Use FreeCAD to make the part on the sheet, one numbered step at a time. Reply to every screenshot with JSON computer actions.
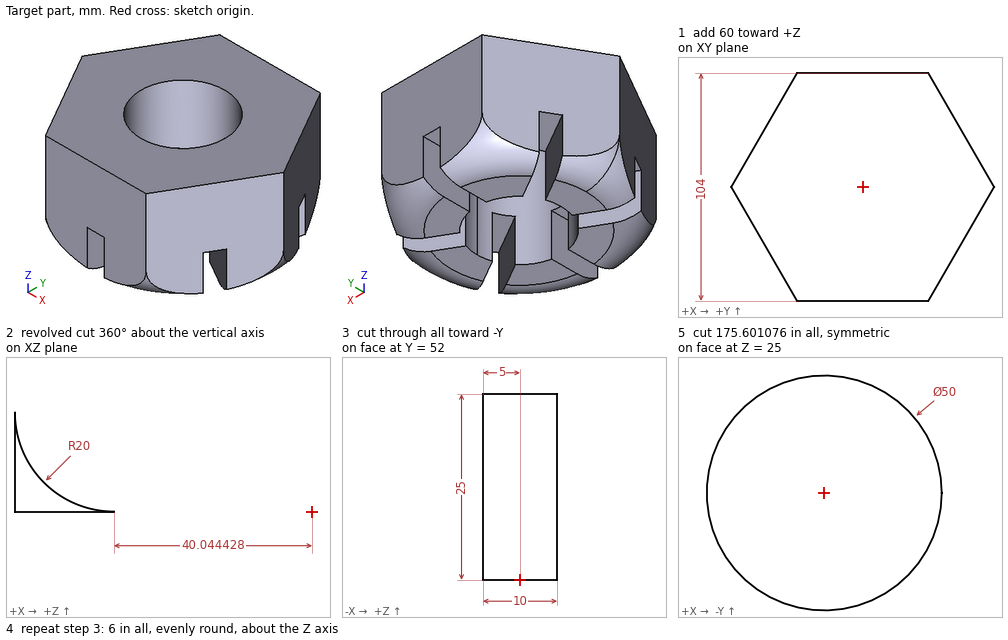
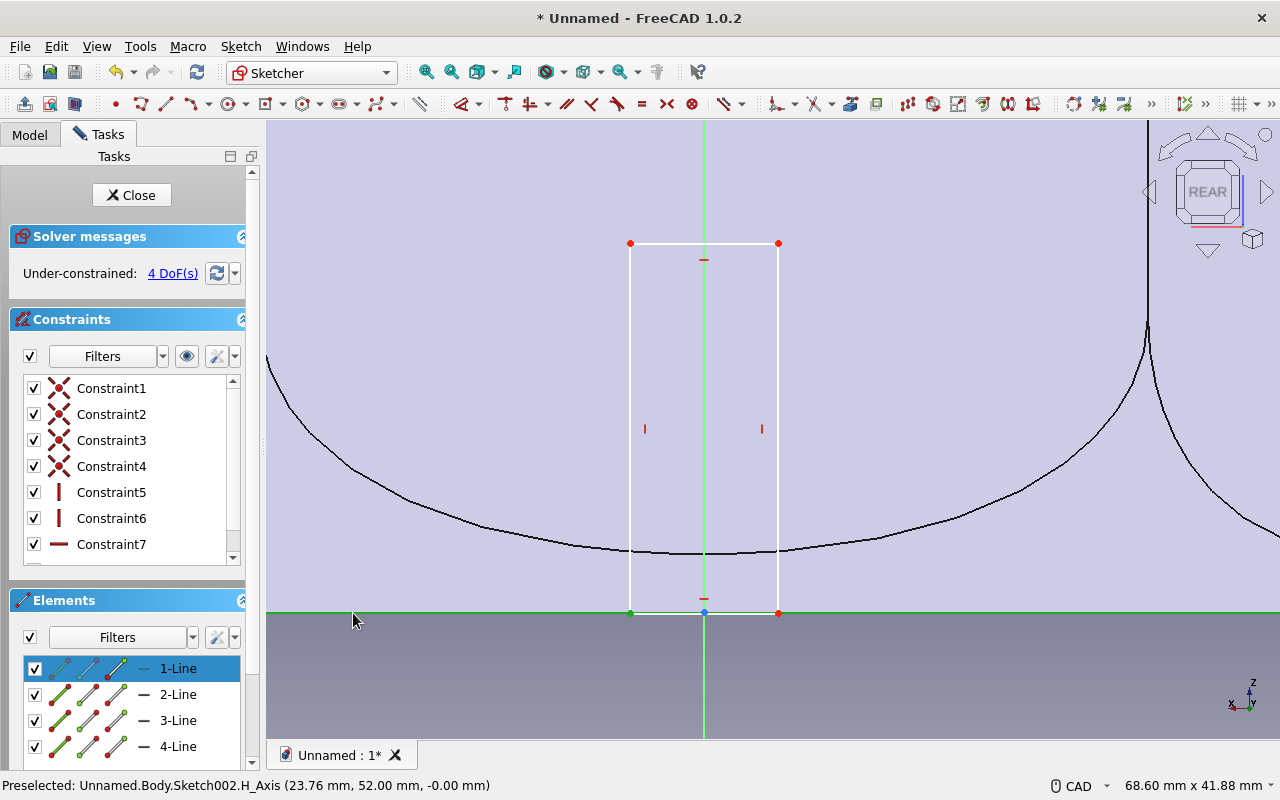
{"action": "left_click", "coordinate": [505, 104]}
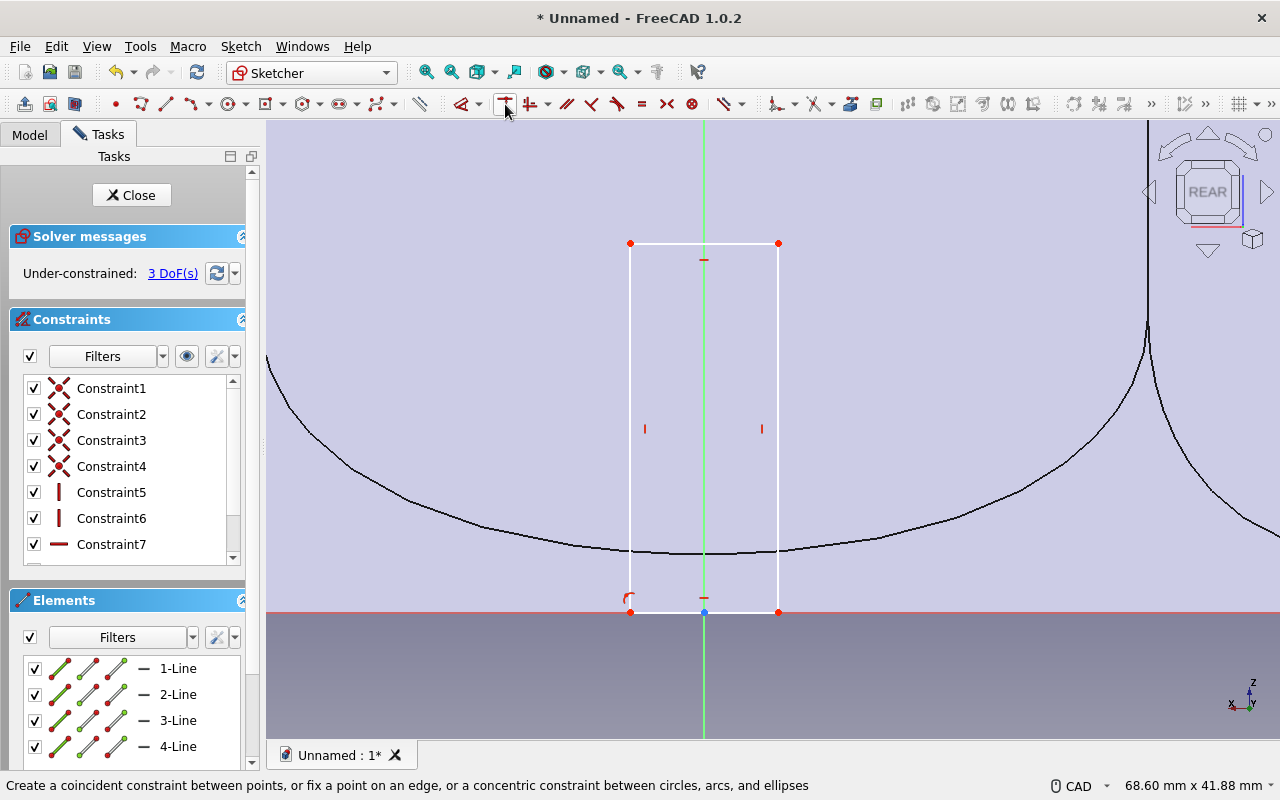
{"action": "key", "text": "d"}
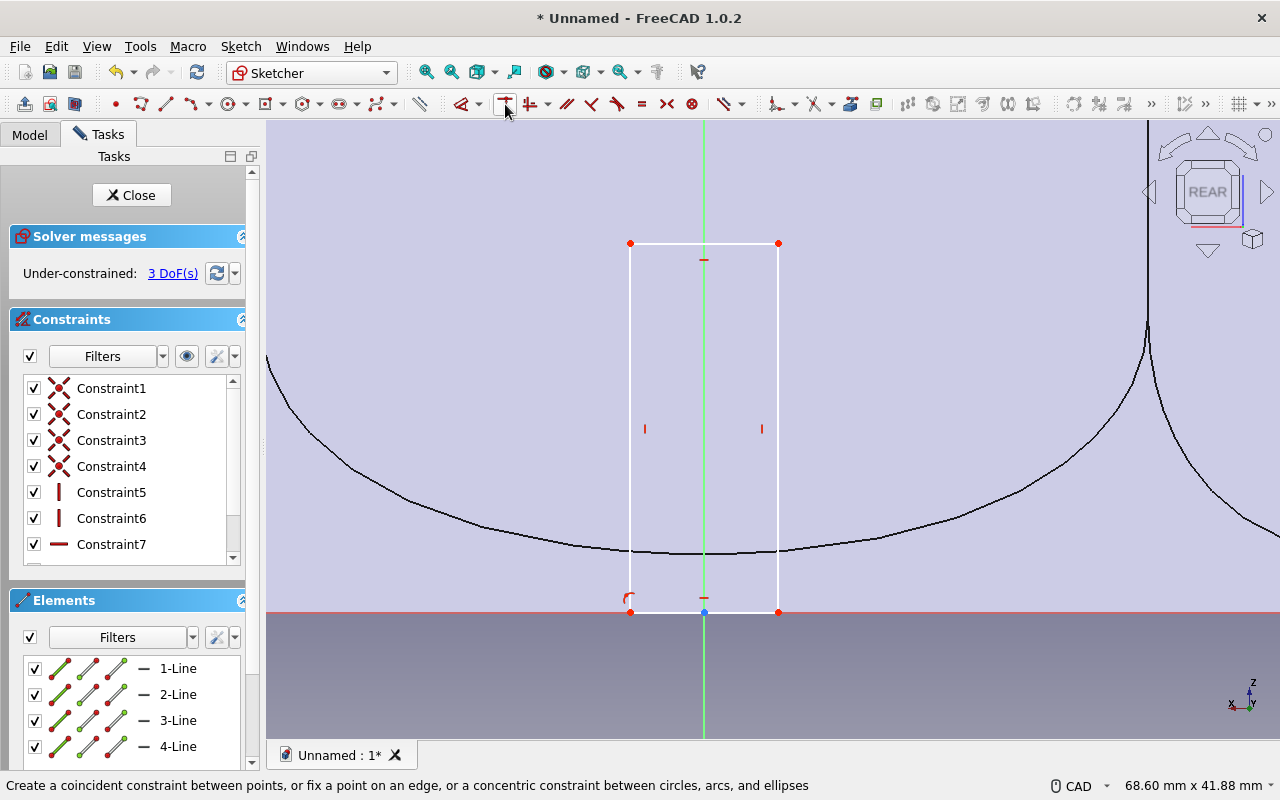
{"action": "left_click", "coordinate": [630, 355]}
{"action": "left_click", "coordinate": [596, 428]}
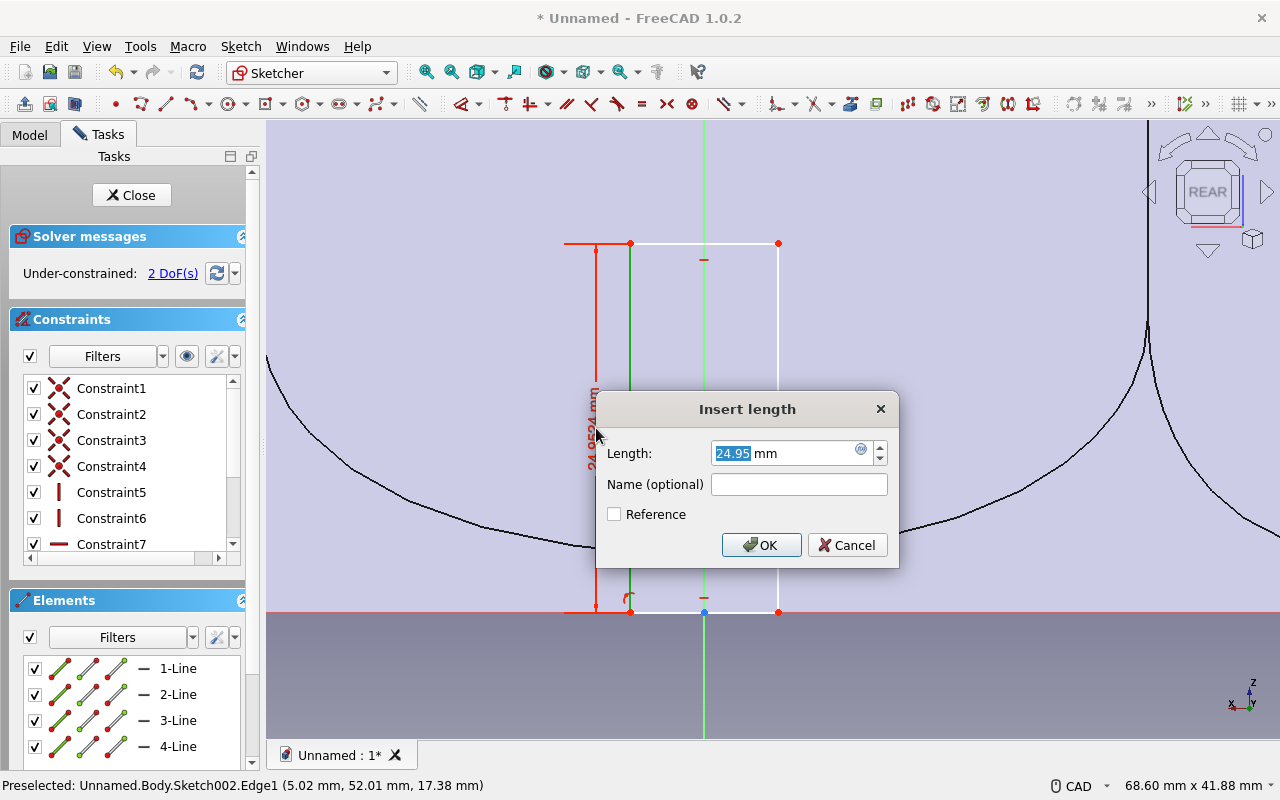
{"action": "type", "text": "25"}
{"action": "key", "text": "Return"}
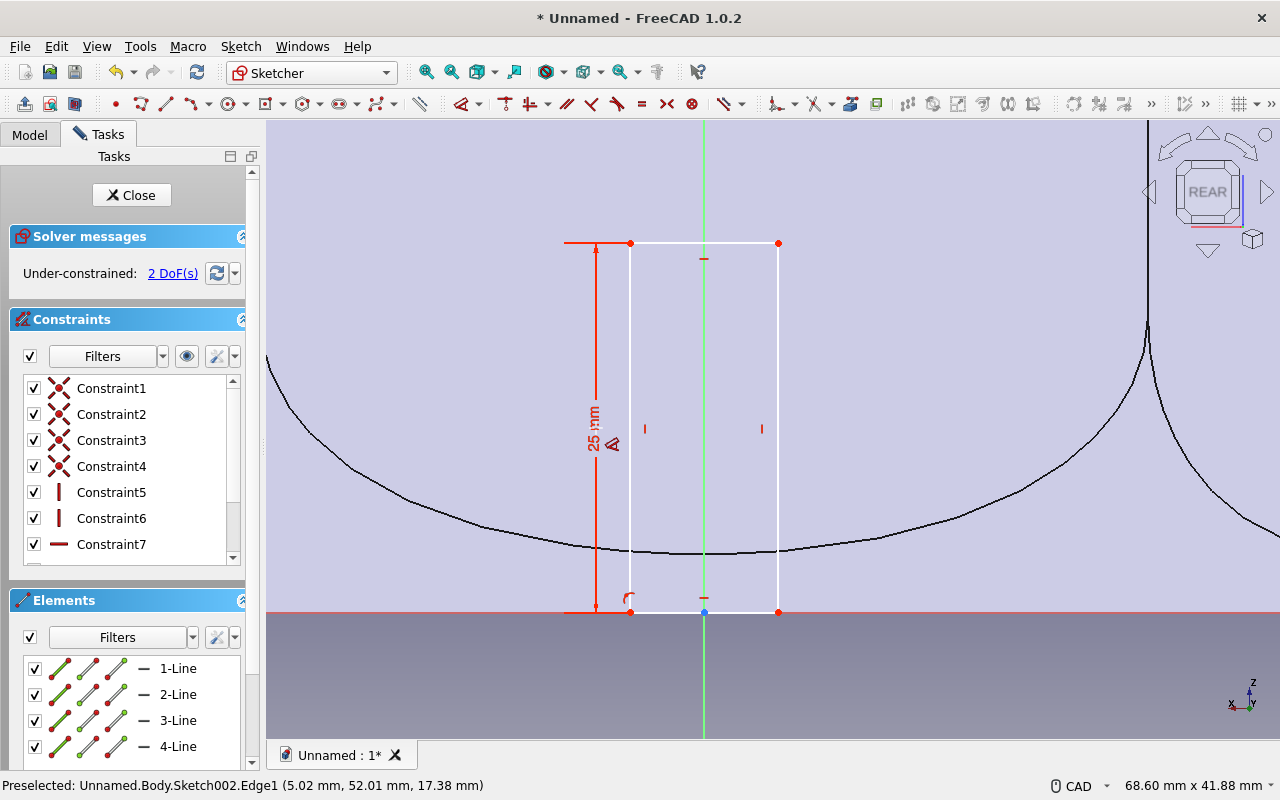
{"action": "left_click", "coordinate": [674, 613]}
{"action": "left_click", "coordinate": [670, 647]}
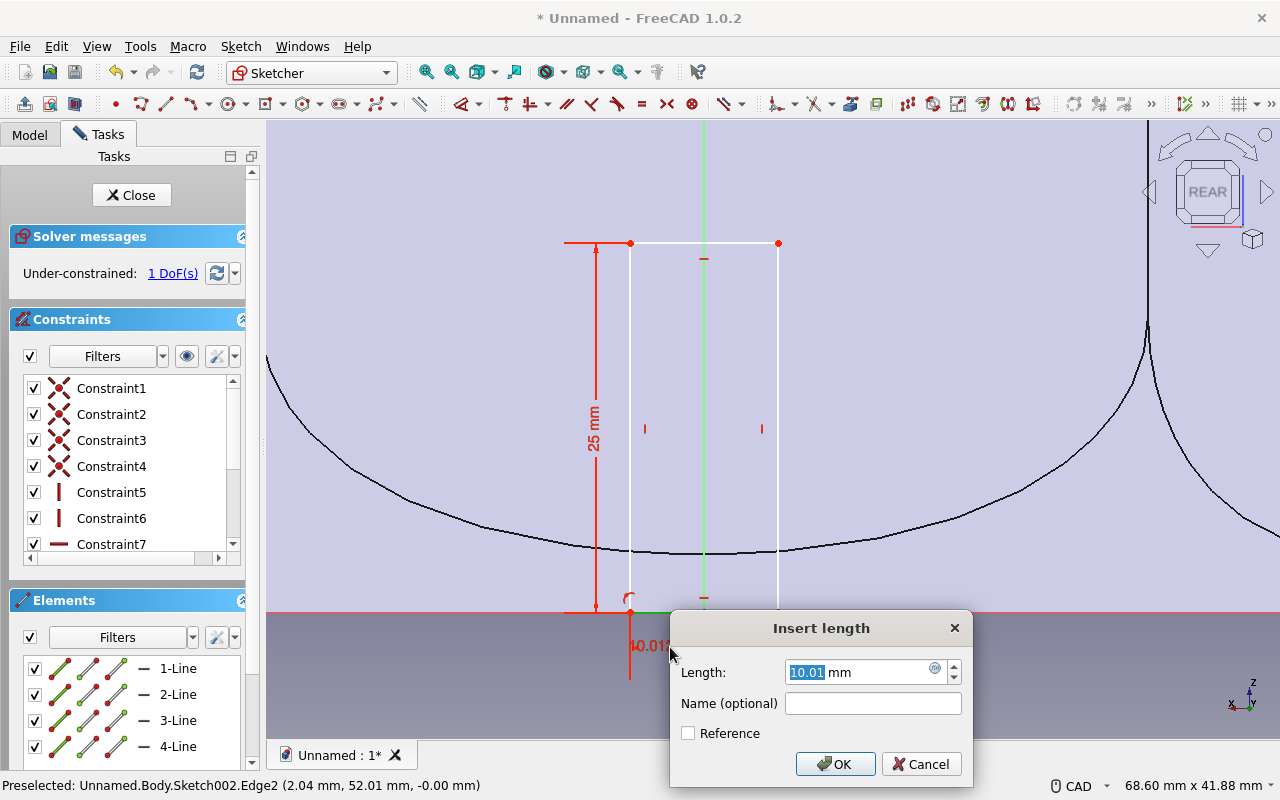
{"action": "type", "text": "10"}
{"action": "key", "text": "Return"}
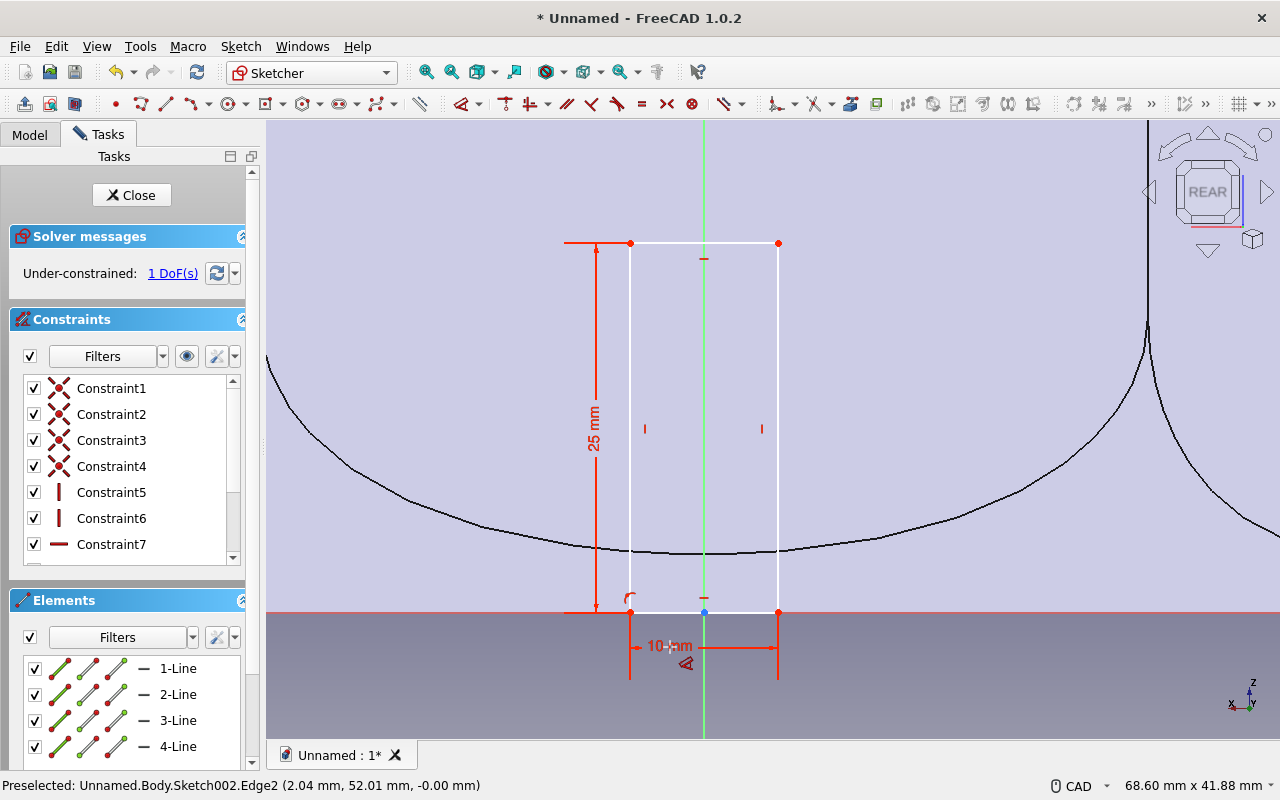
{"action": "left_click", "coordinate": [630, 243]}
{"action": "left_click", "coordinate": [667, 209]}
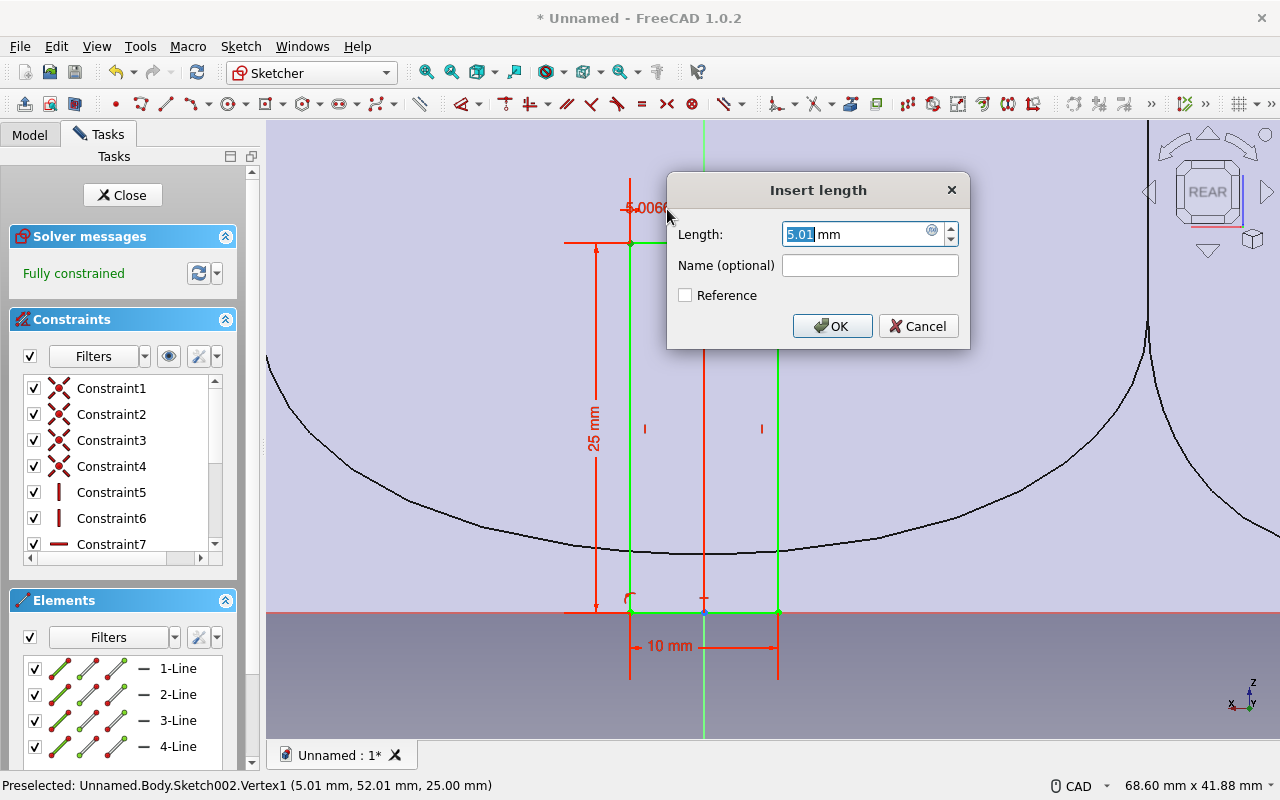
{"action": "type", "text": "5"}
{"action": "key", "text": "Return"}
{"action": "key", "text": "Escape"}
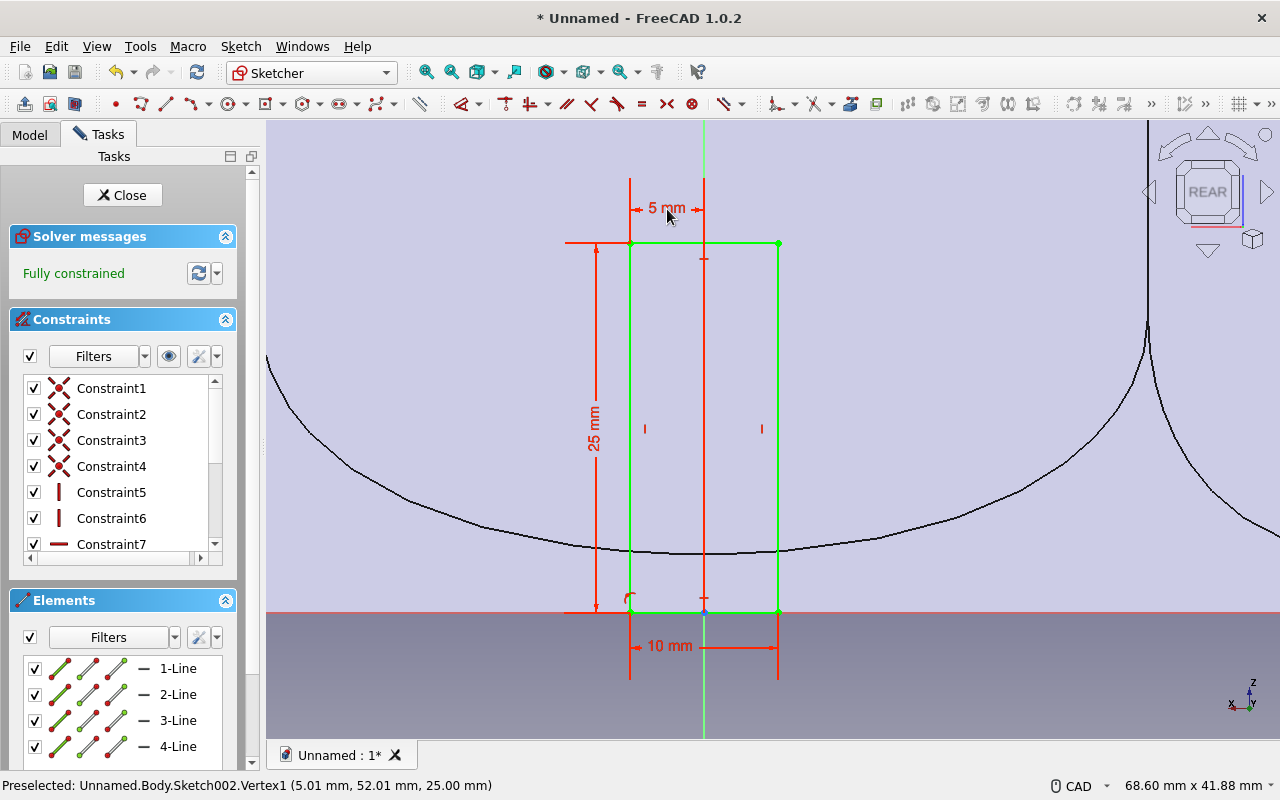
{"action": "left_click", "coordinate": [123, 195]}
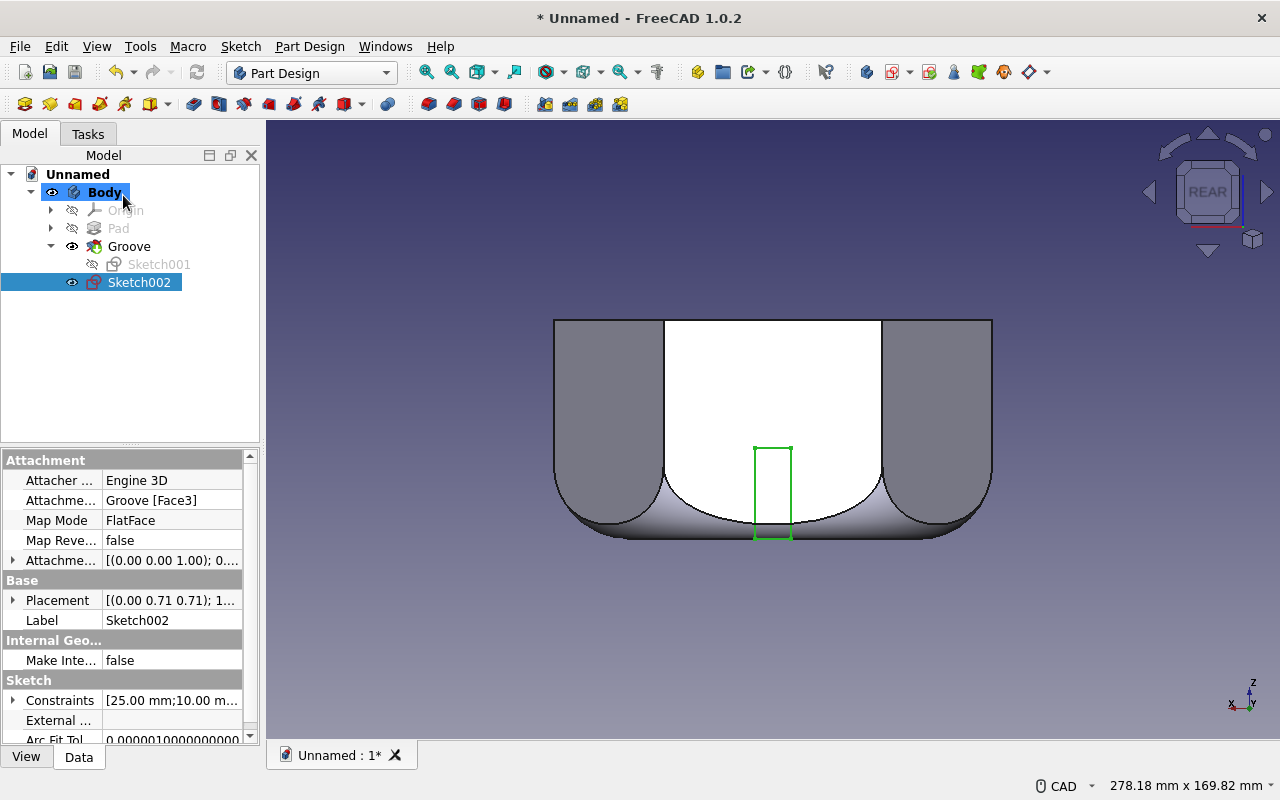
{"action": "left_click", "coordinate": [194, 104]}